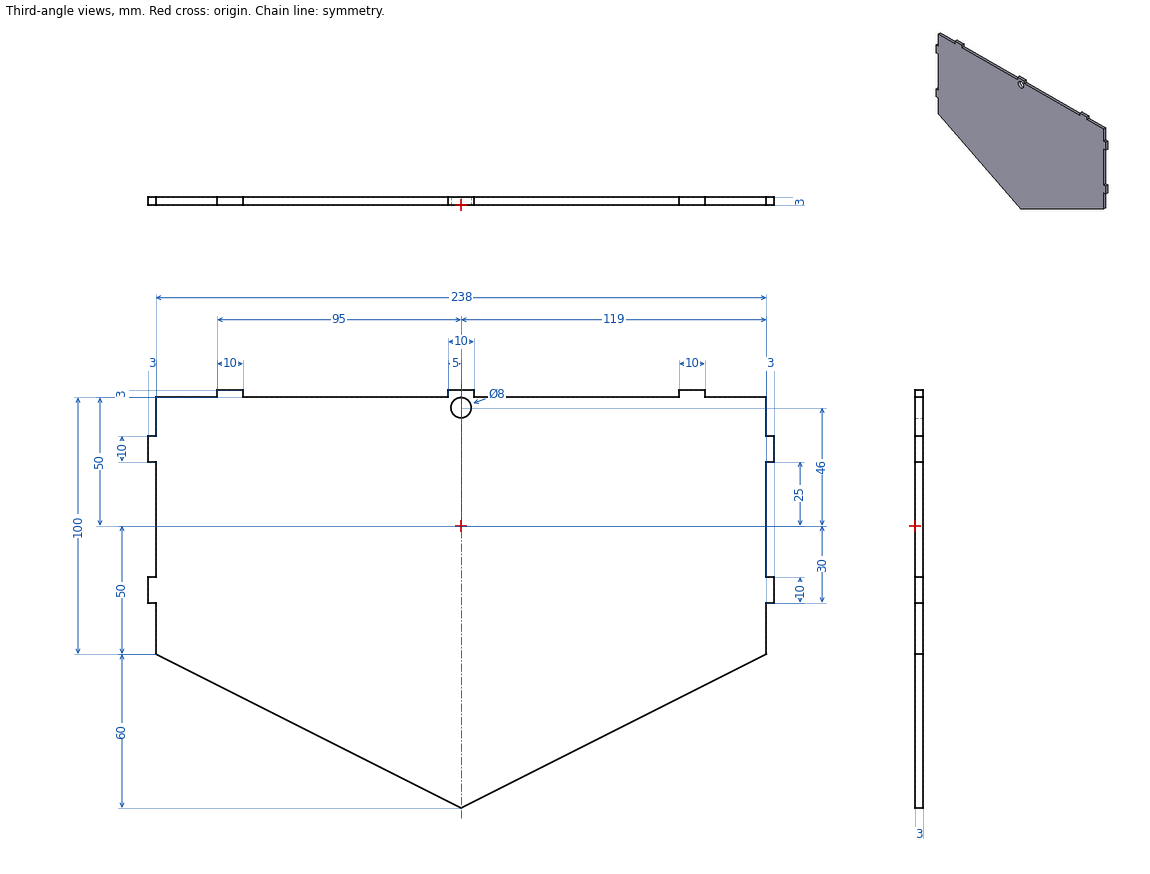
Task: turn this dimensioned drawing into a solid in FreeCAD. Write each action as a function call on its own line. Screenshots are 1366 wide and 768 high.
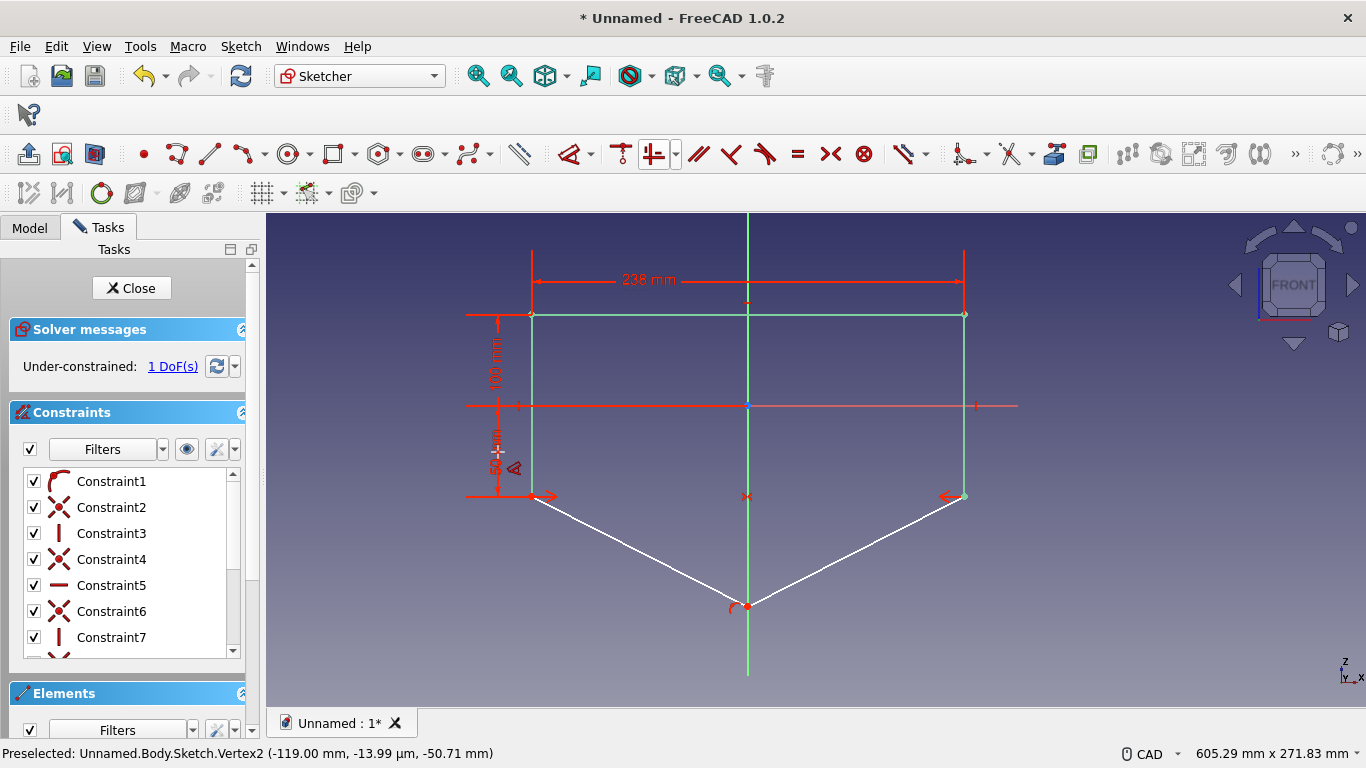
click(683, 574)
click(498, 552)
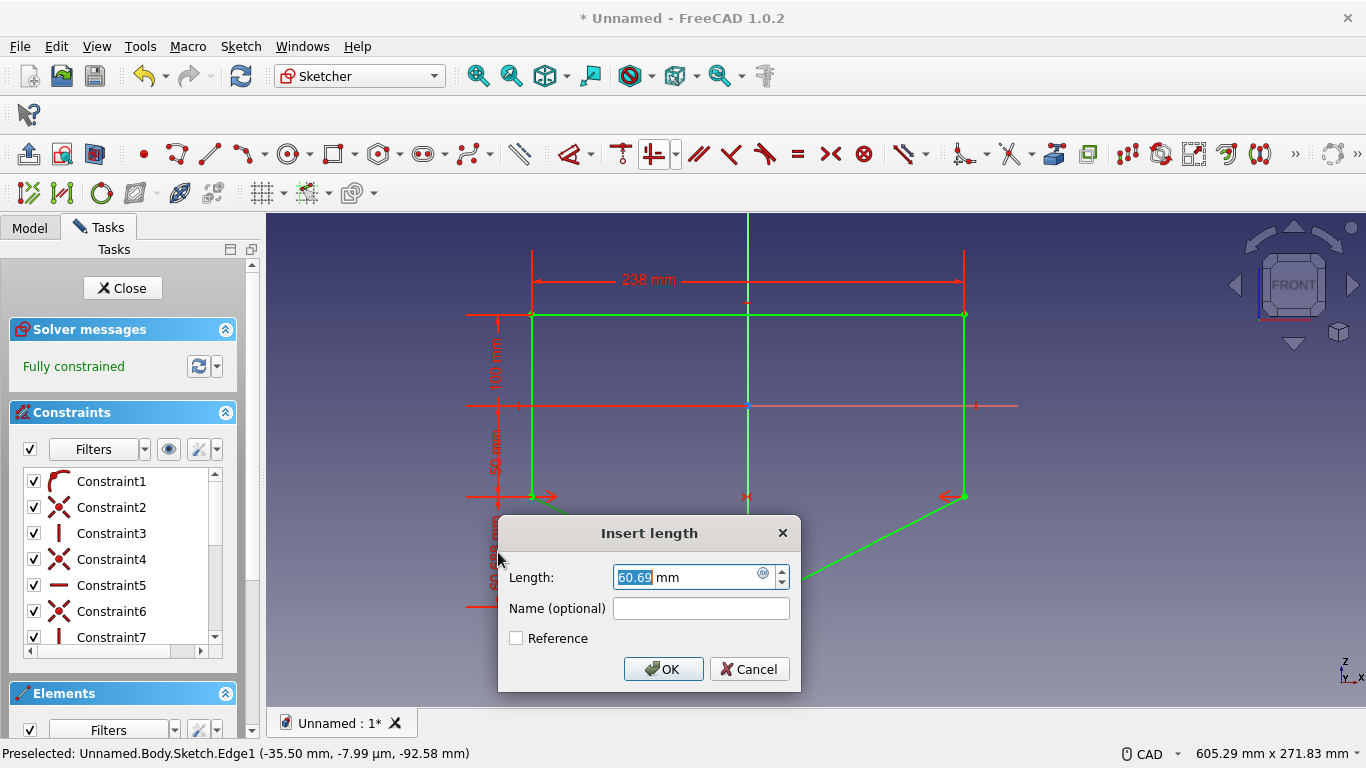
text(60)
key(Return)
key(Escape)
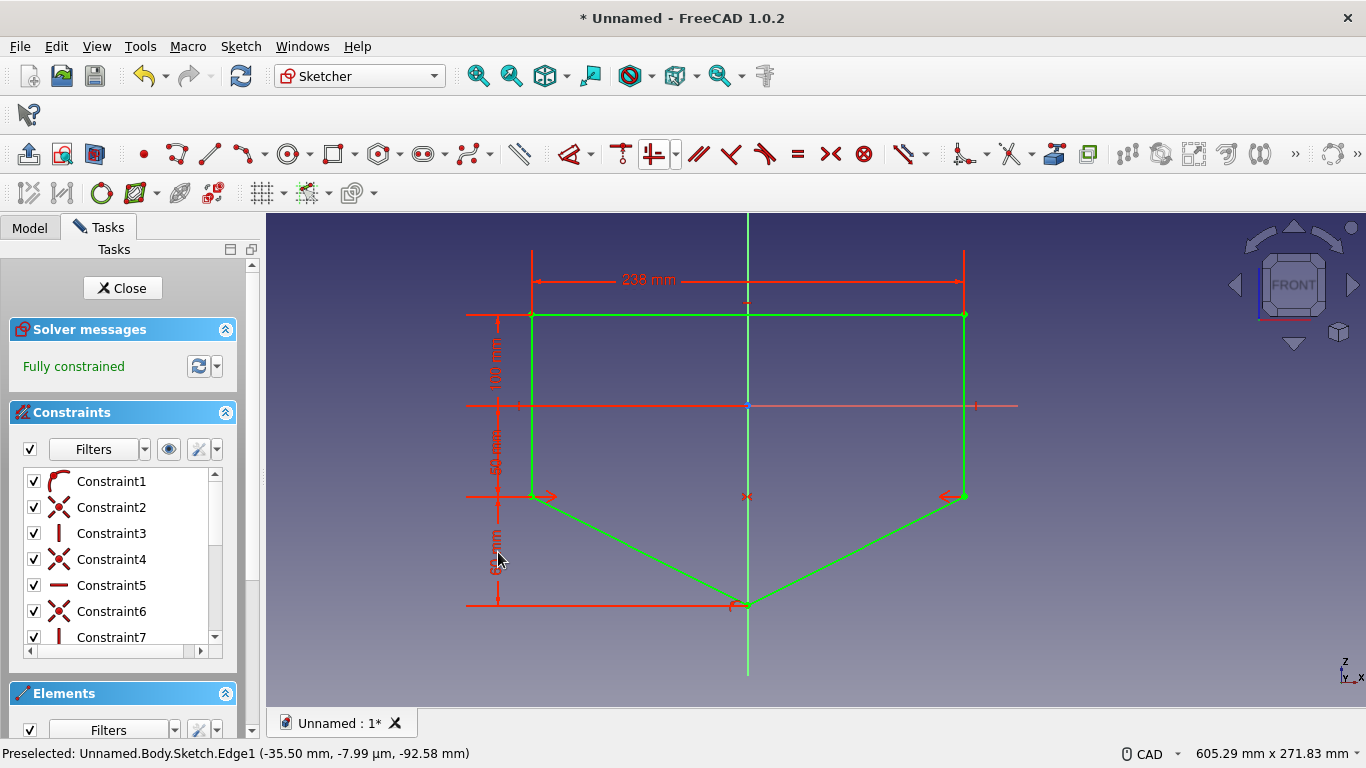
click(123, 288)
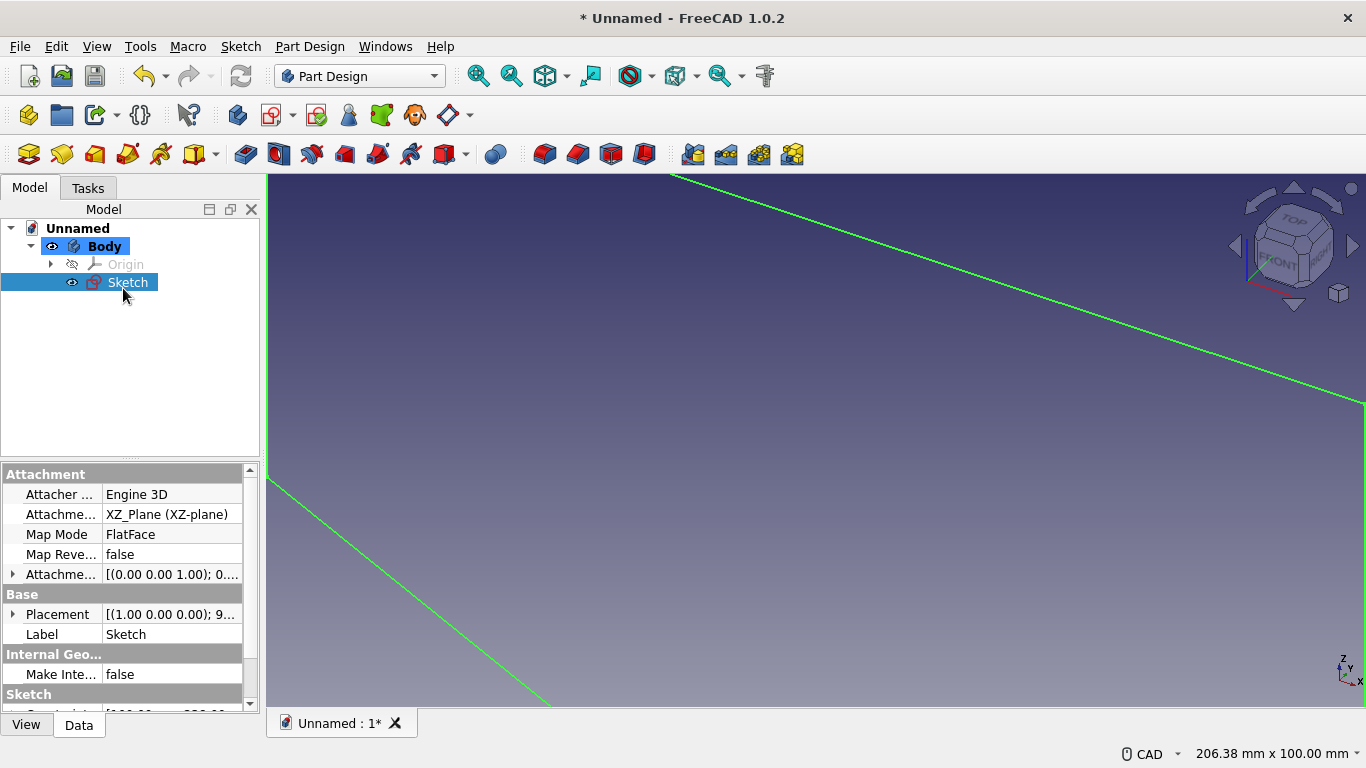
click(29, 154)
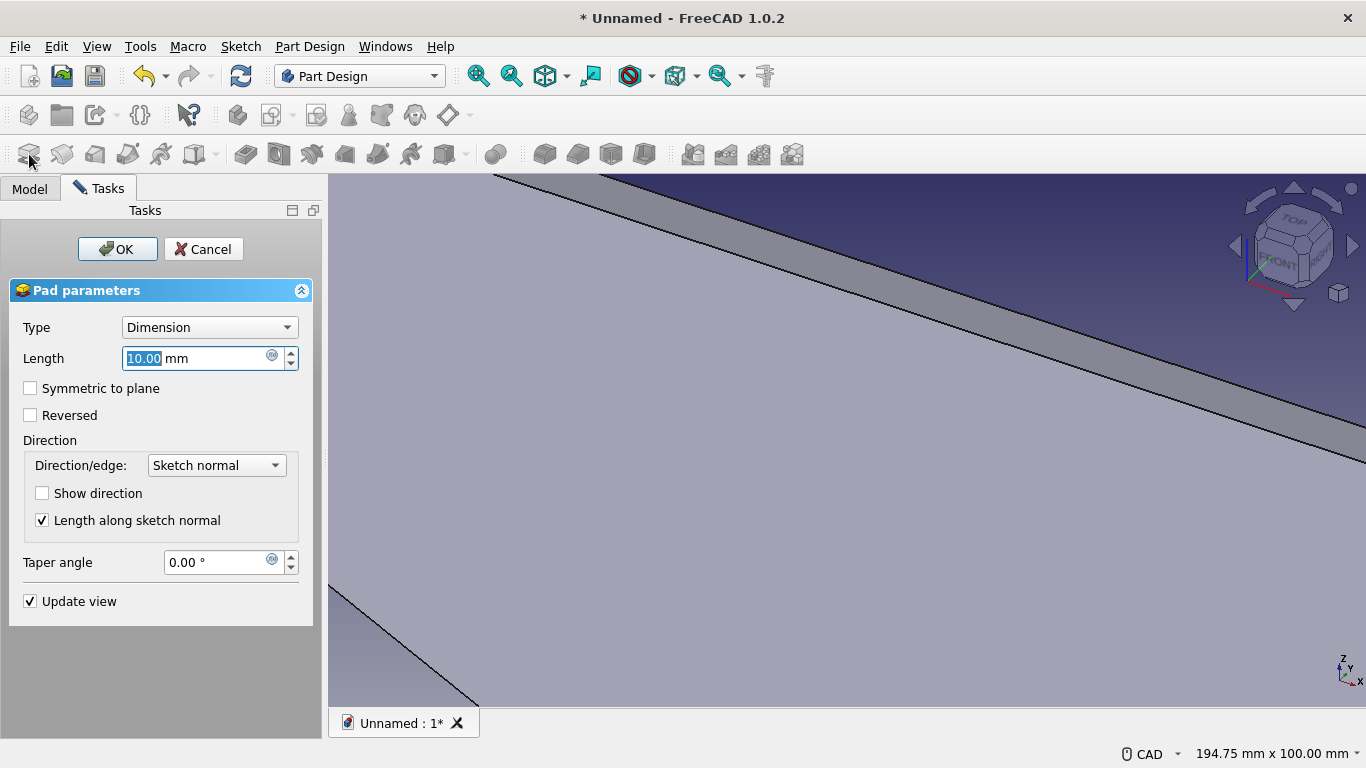
text(3)
key(Tab)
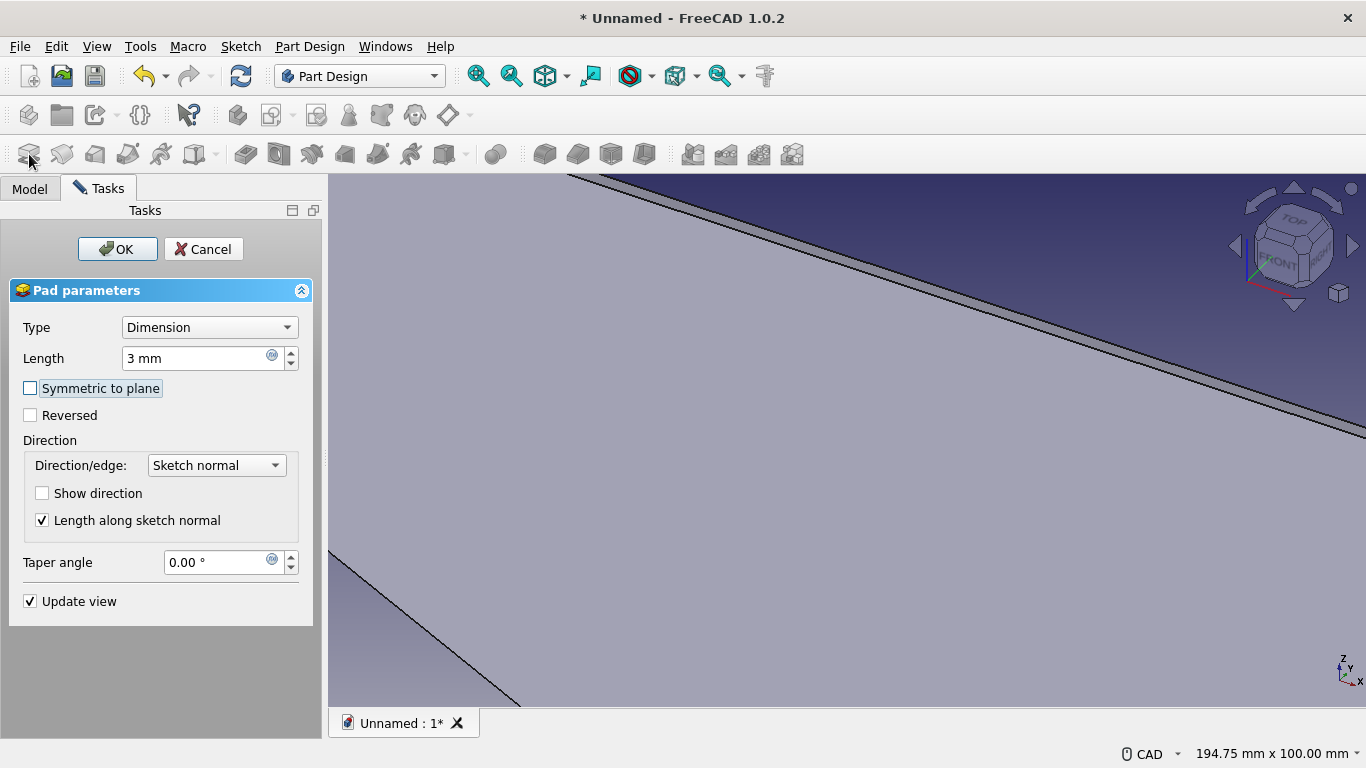
click(31, 415)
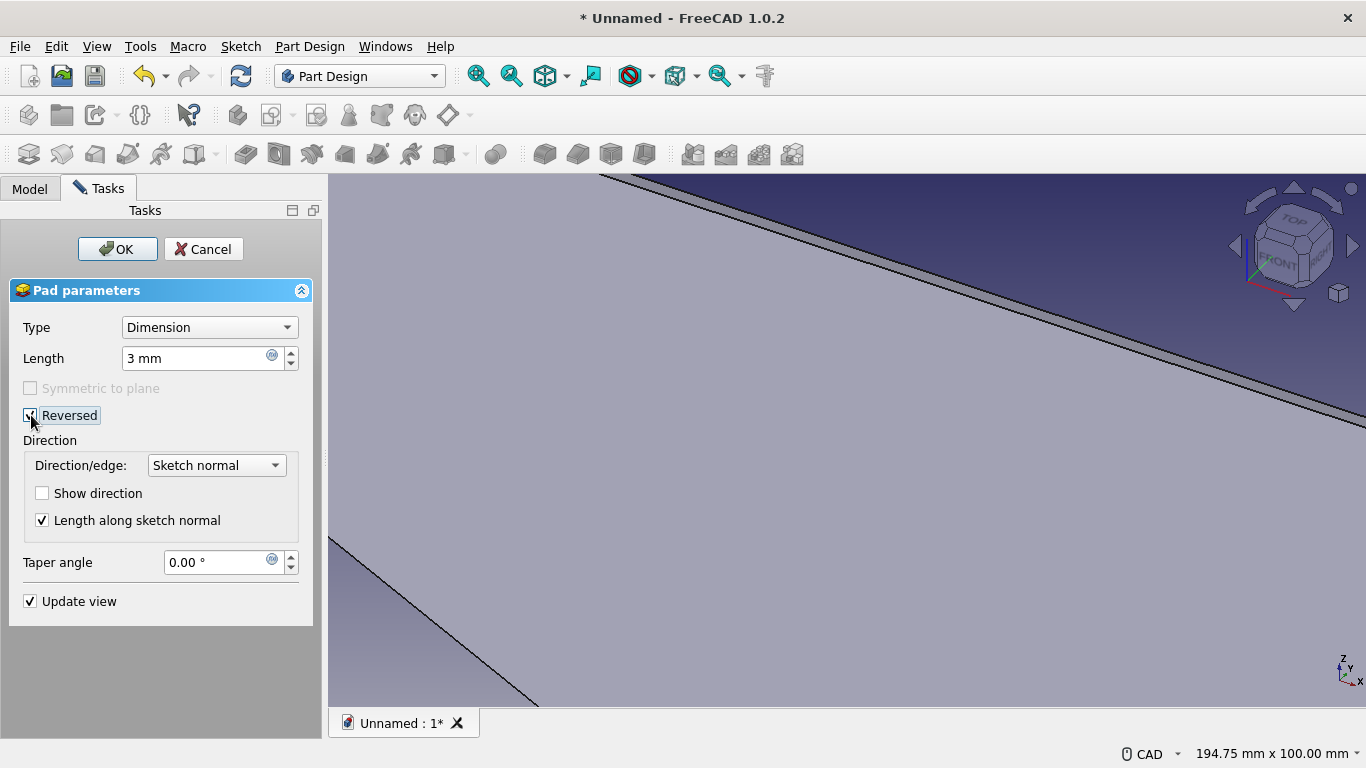
click(118, 249)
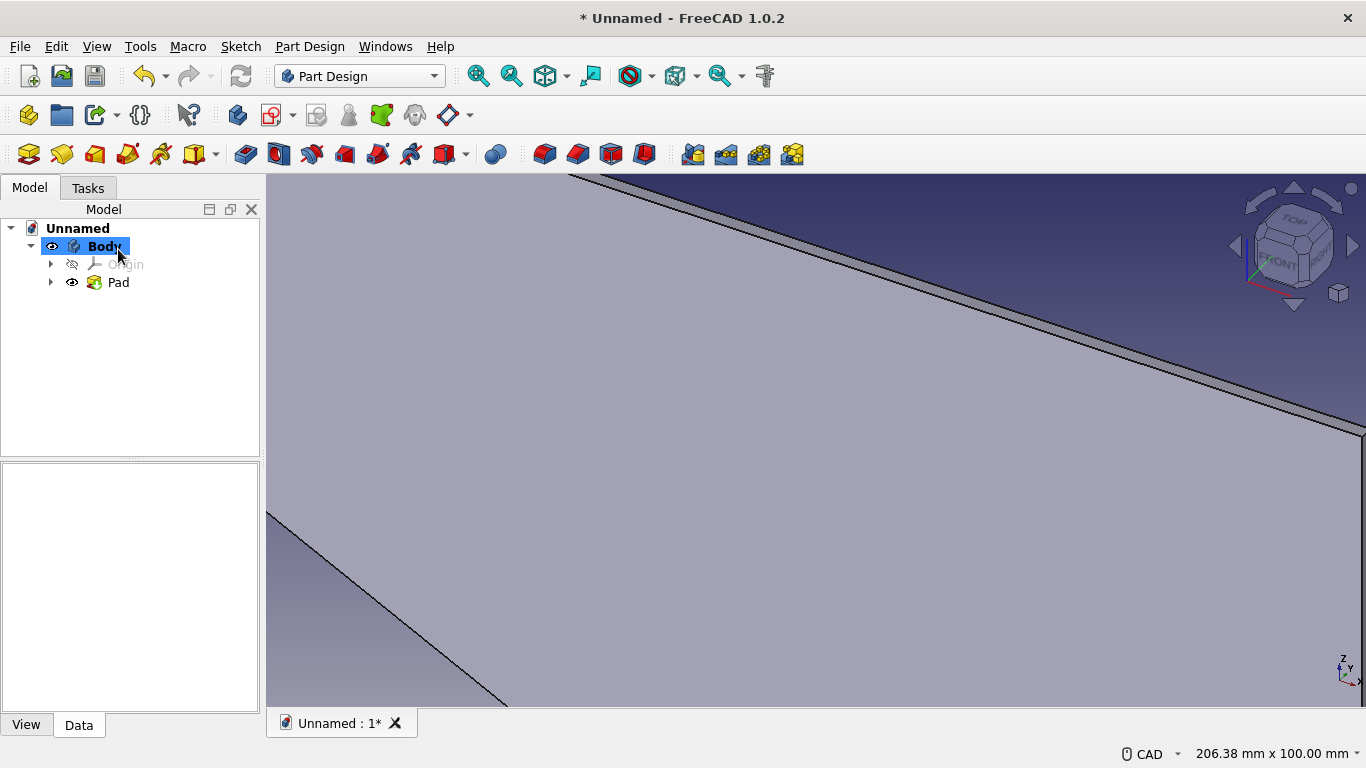
click(479, 76)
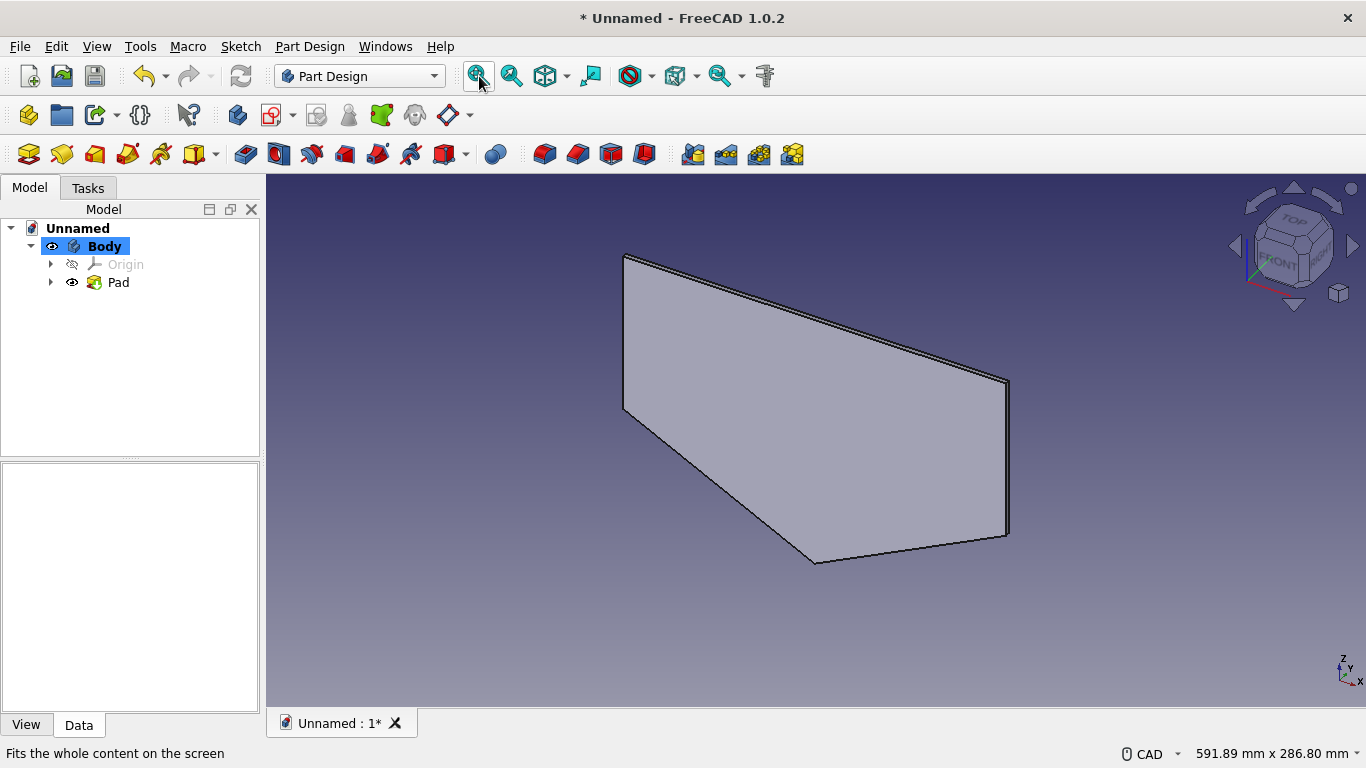
key(4)